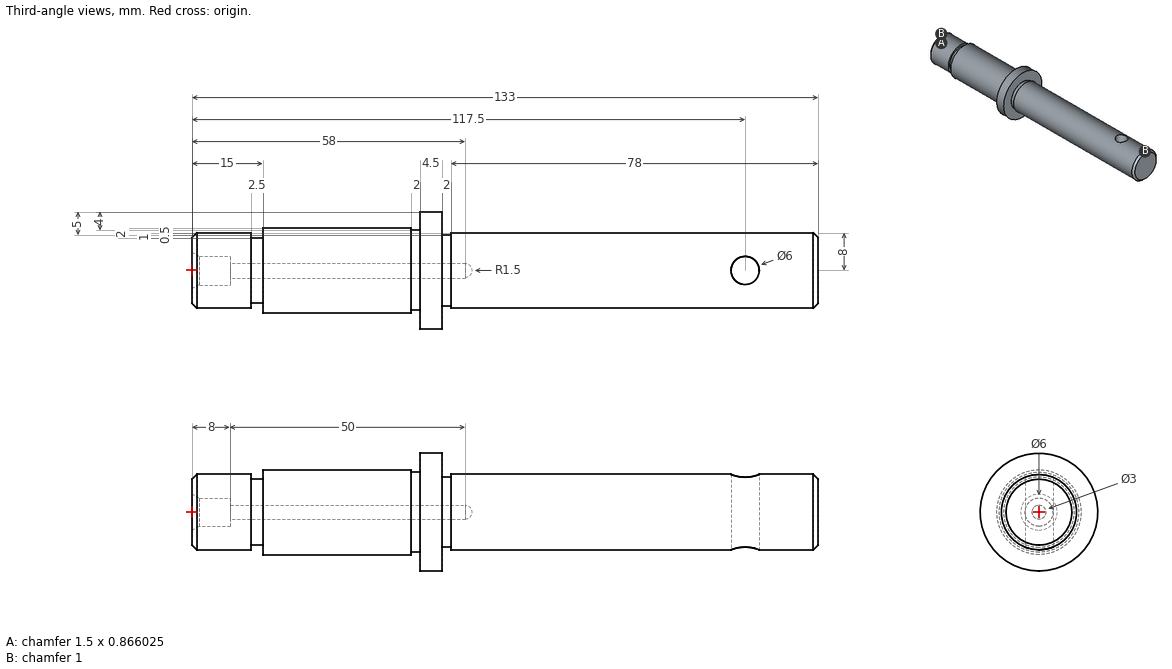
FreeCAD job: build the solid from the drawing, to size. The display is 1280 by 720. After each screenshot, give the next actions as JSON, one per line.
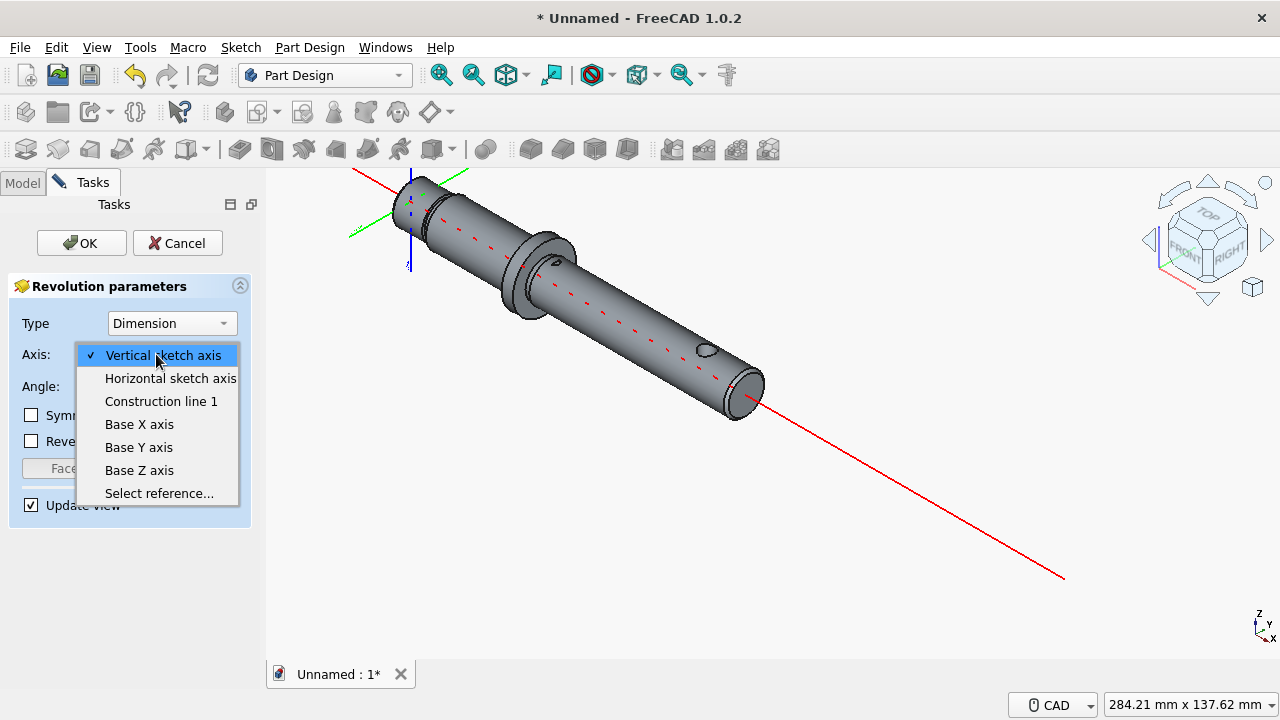
{"action": "left_click", "coordinate": [156, 402]}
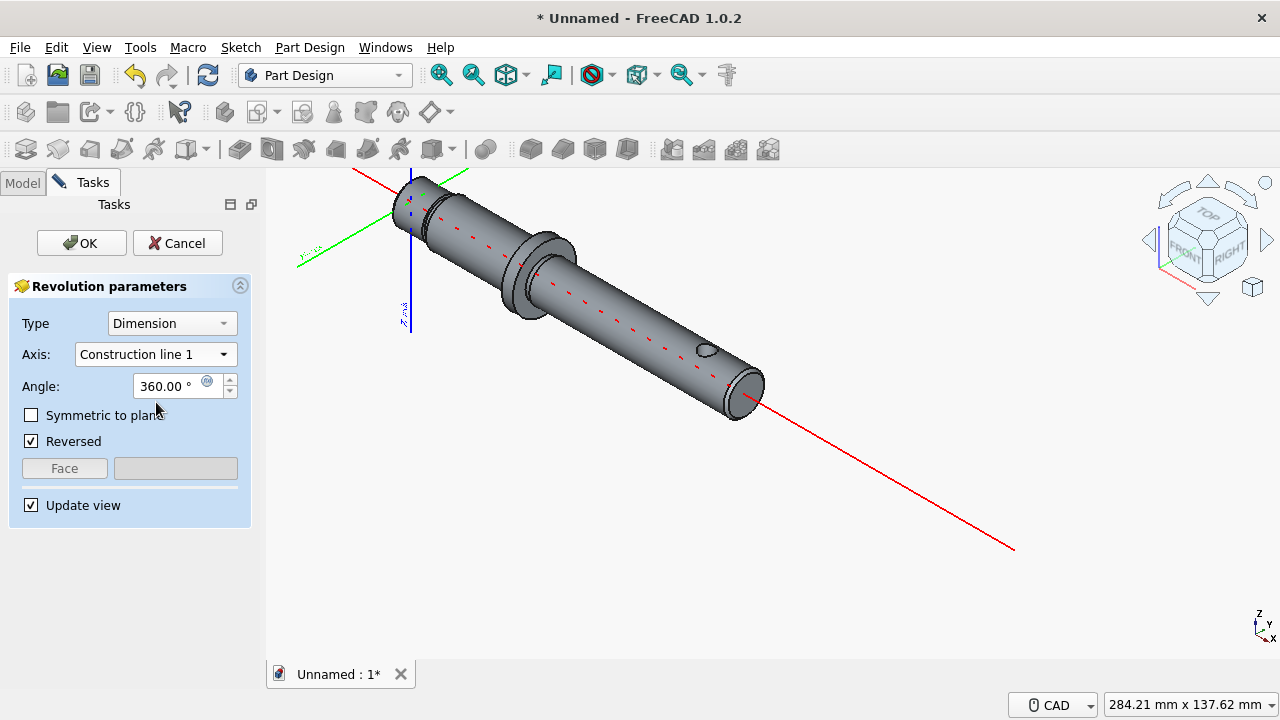
{"action": "left_click", "coordinate": [82, 243]}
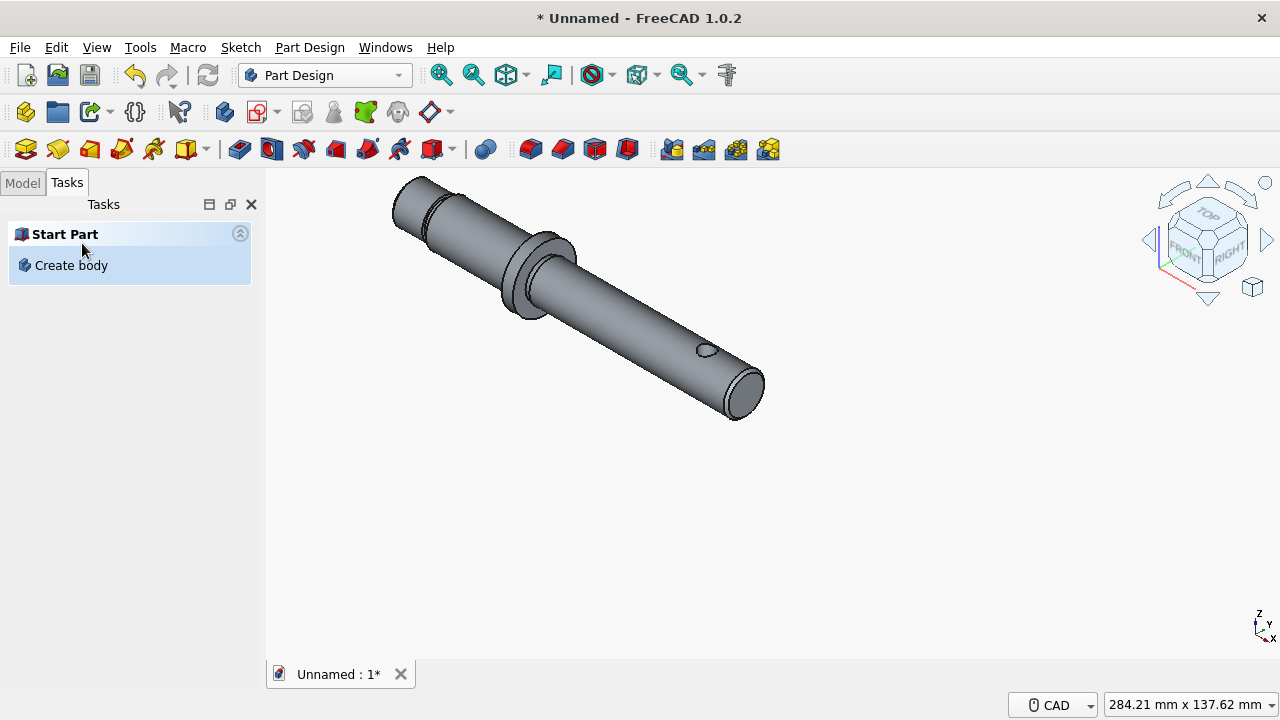
{"action": "key", "text": "v f"}